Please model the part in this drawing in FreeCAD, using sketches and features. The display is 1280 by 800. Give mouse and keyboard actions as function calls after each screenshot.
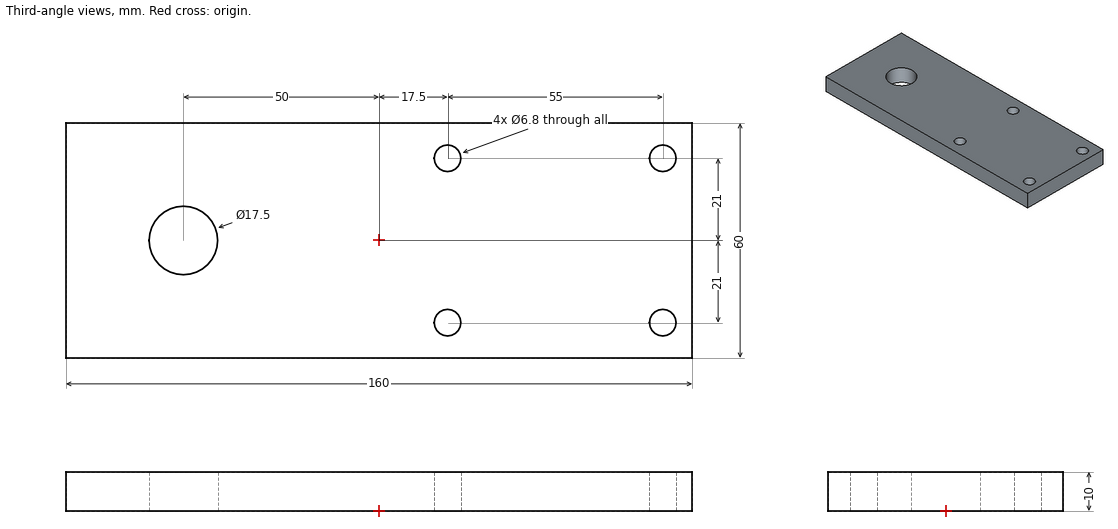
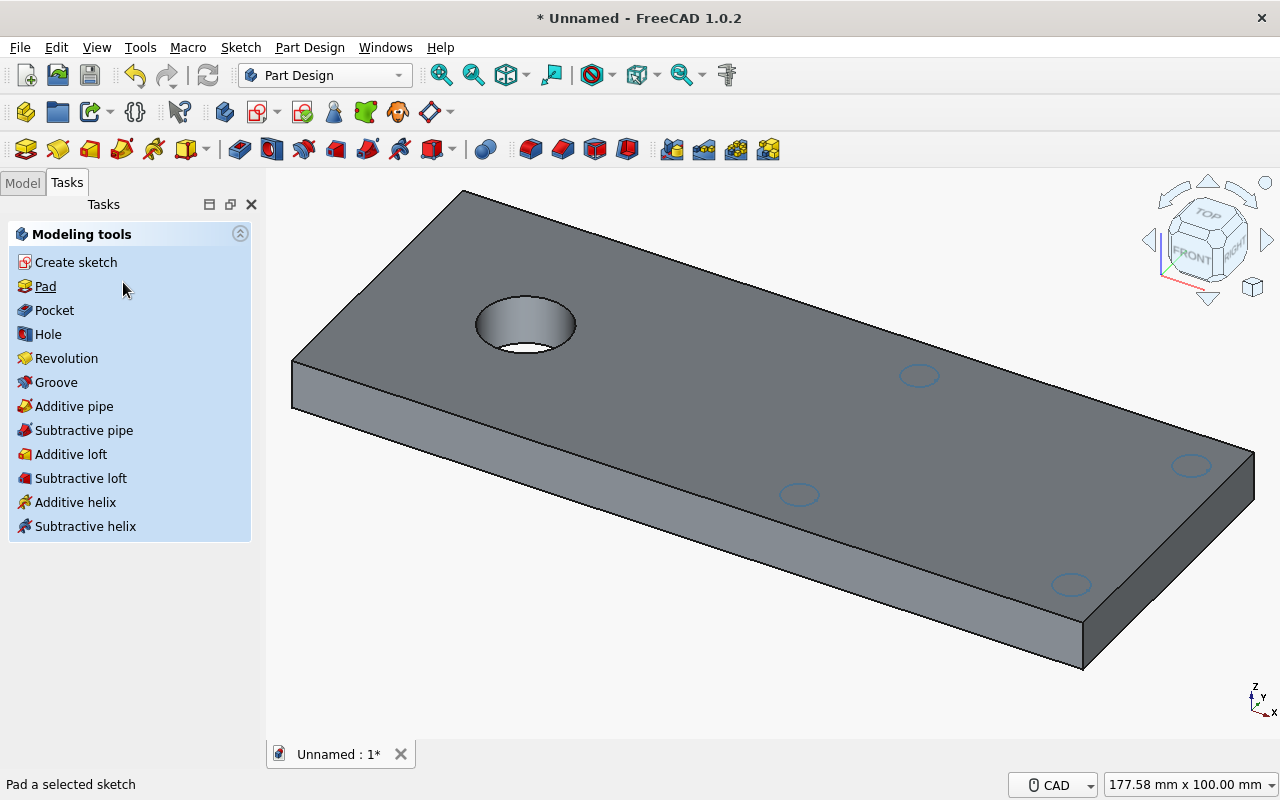
click(272, 150)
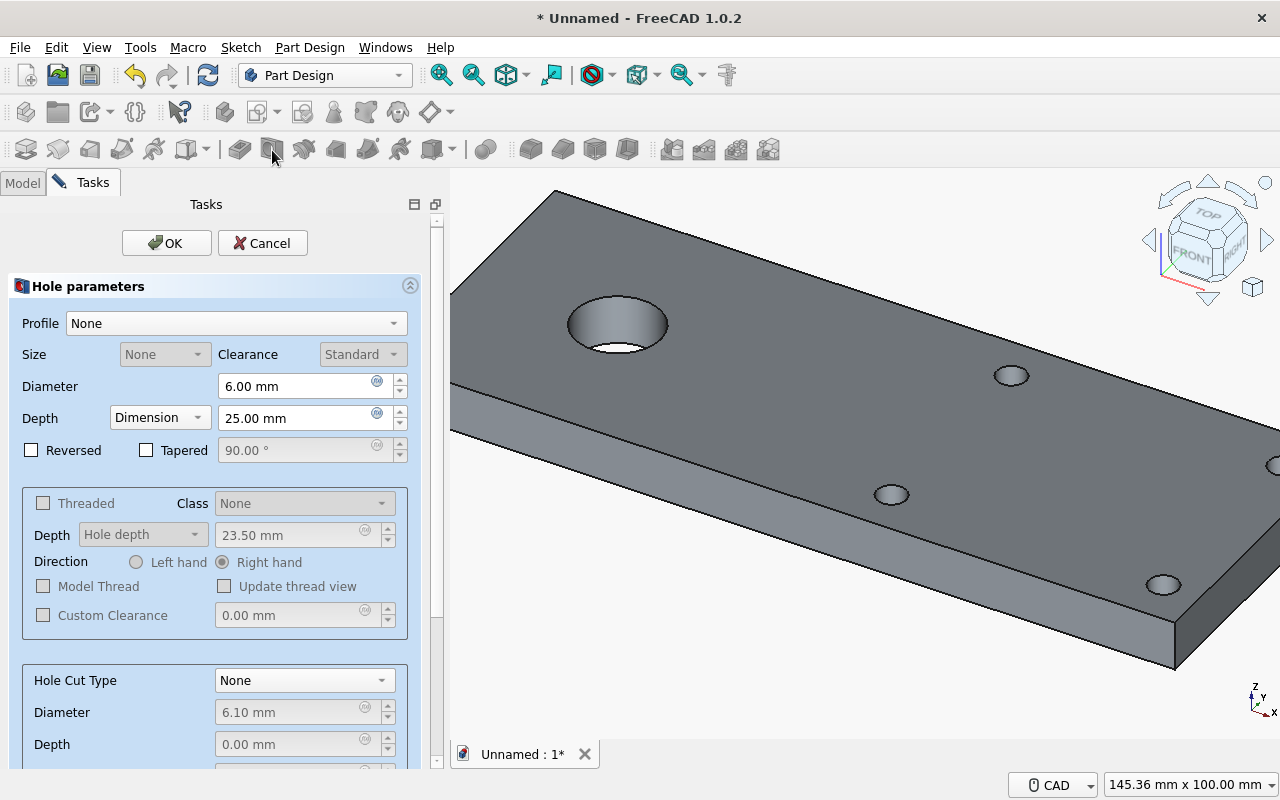
triple_click(305, 386)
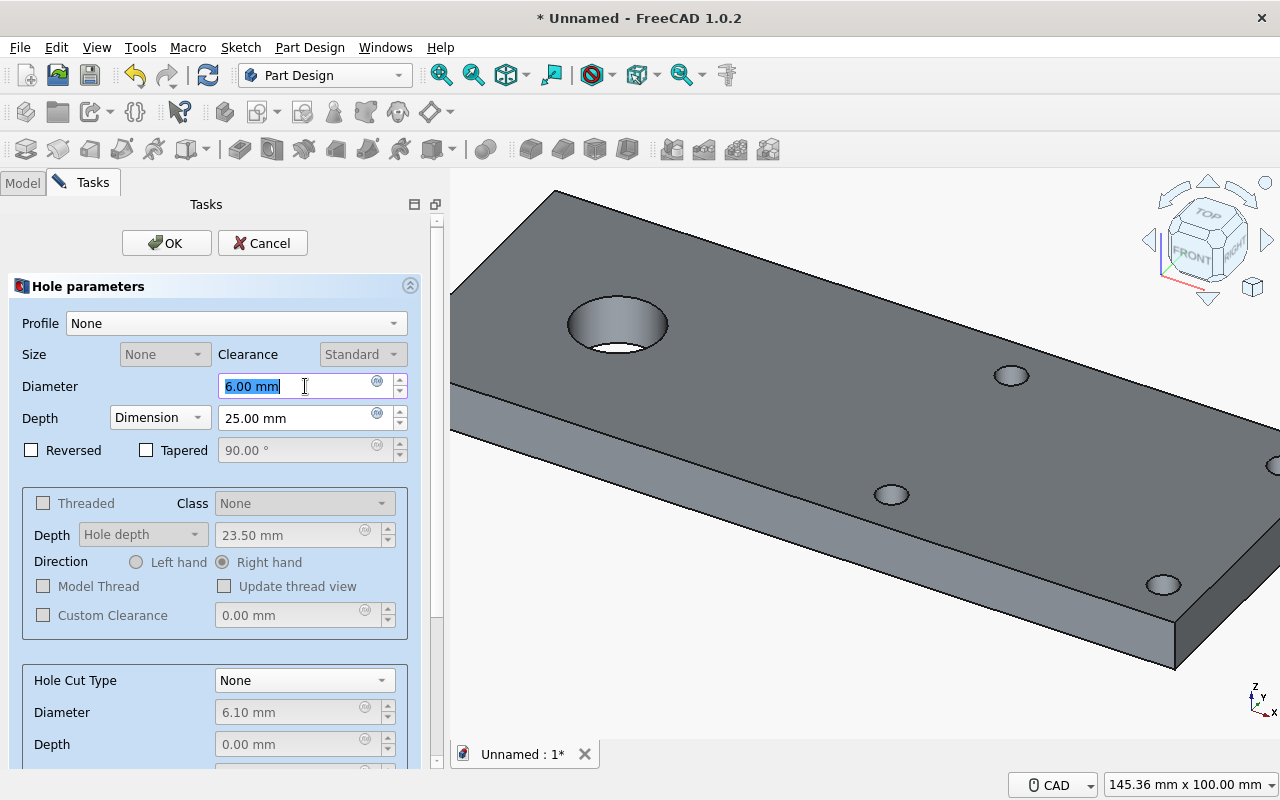
text(6.8)
key(Tab)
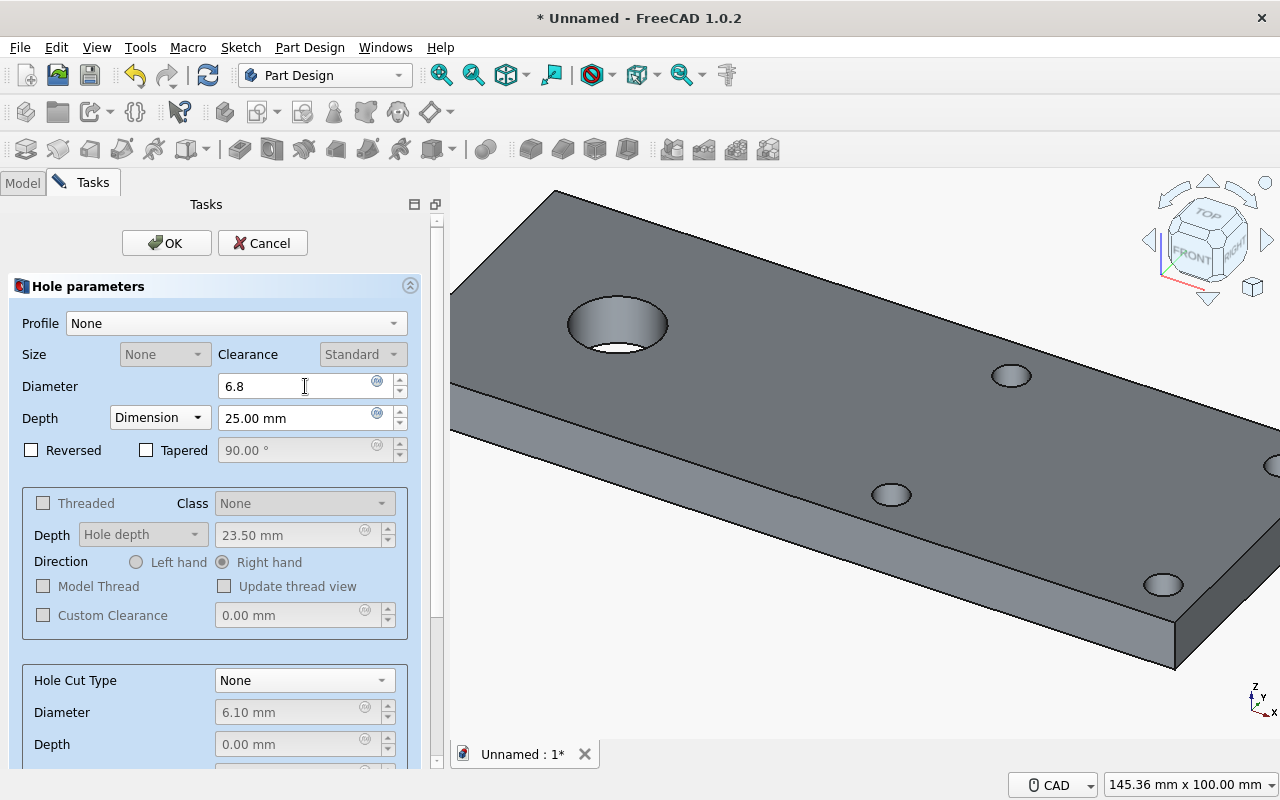
click(161, 418)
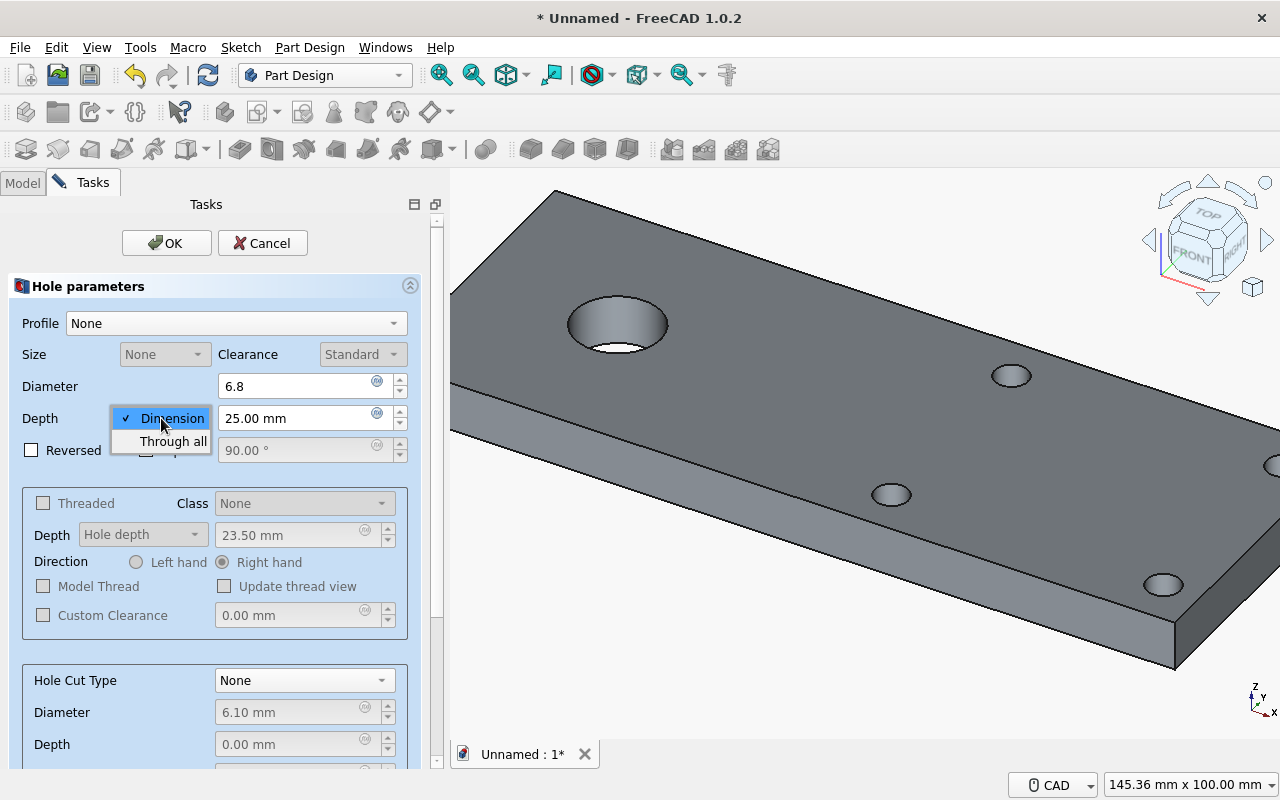
click(160, 442)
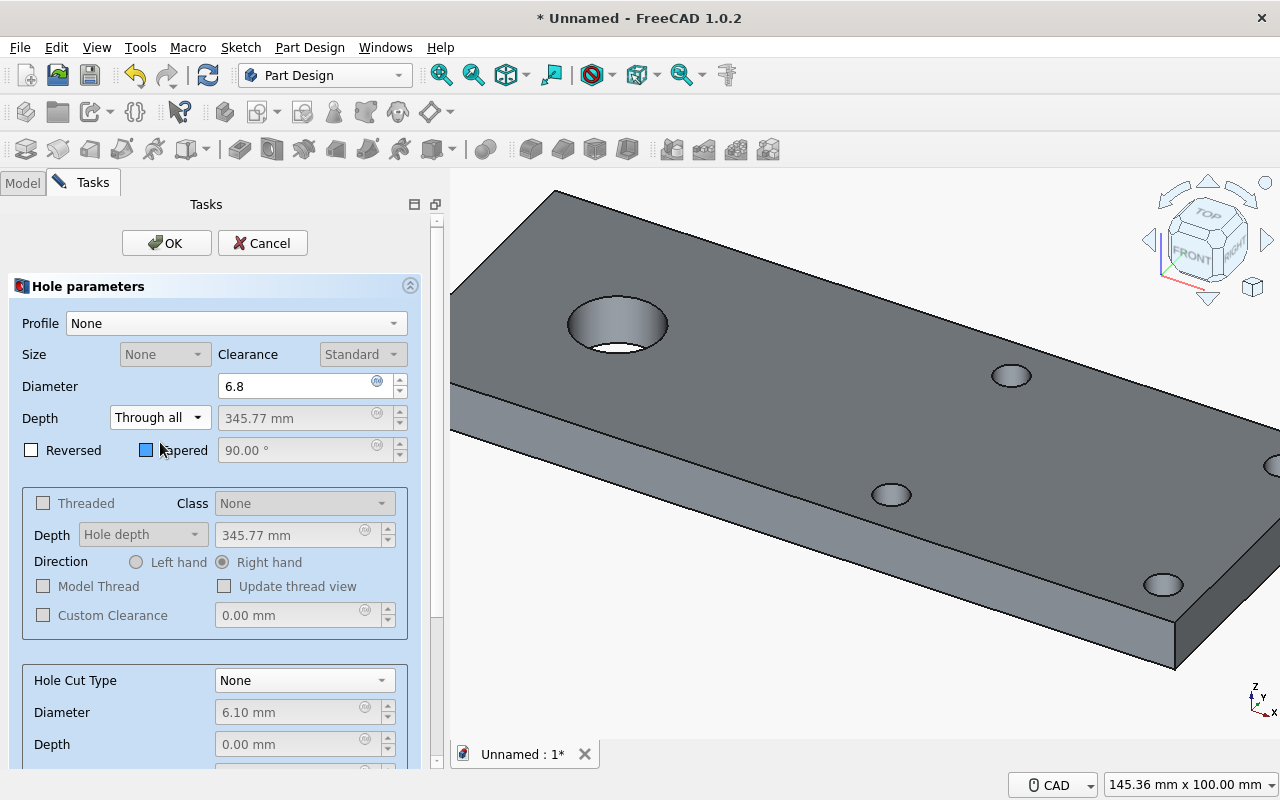
click(167, 243)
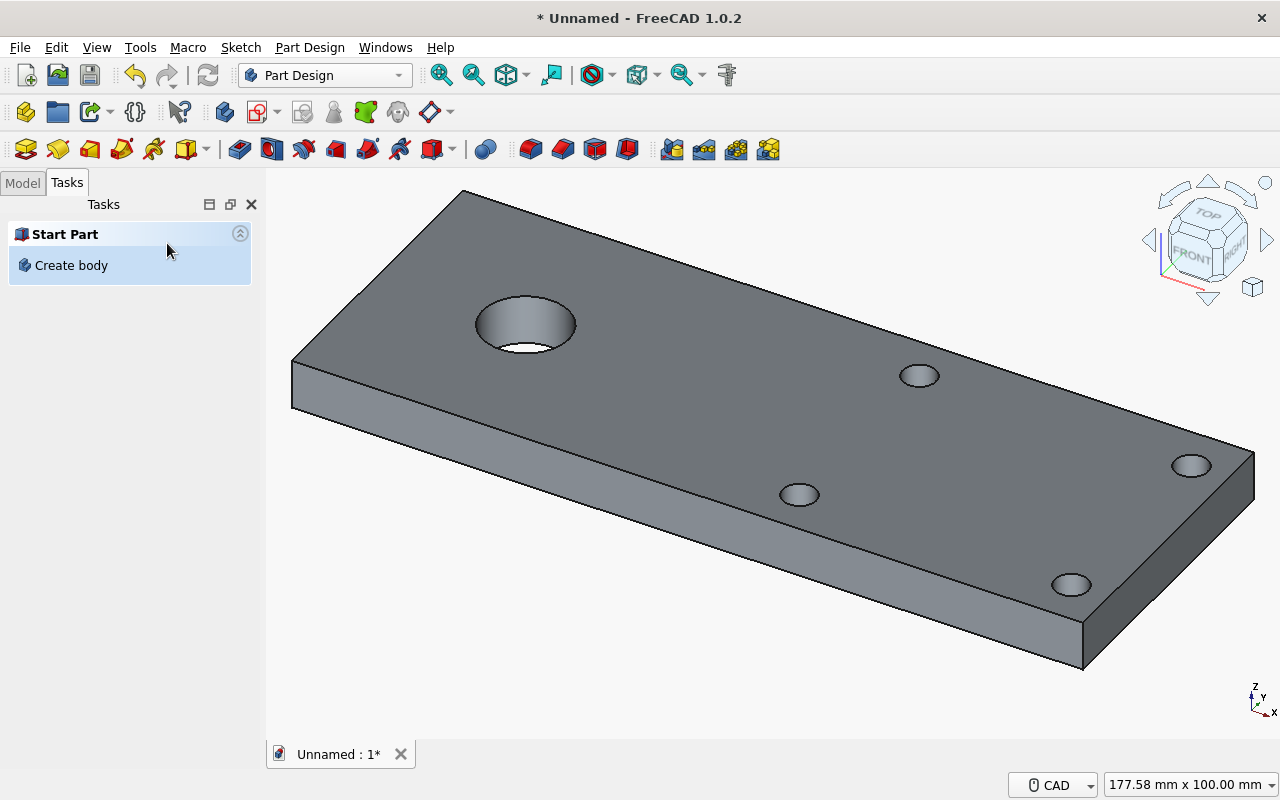
key(0)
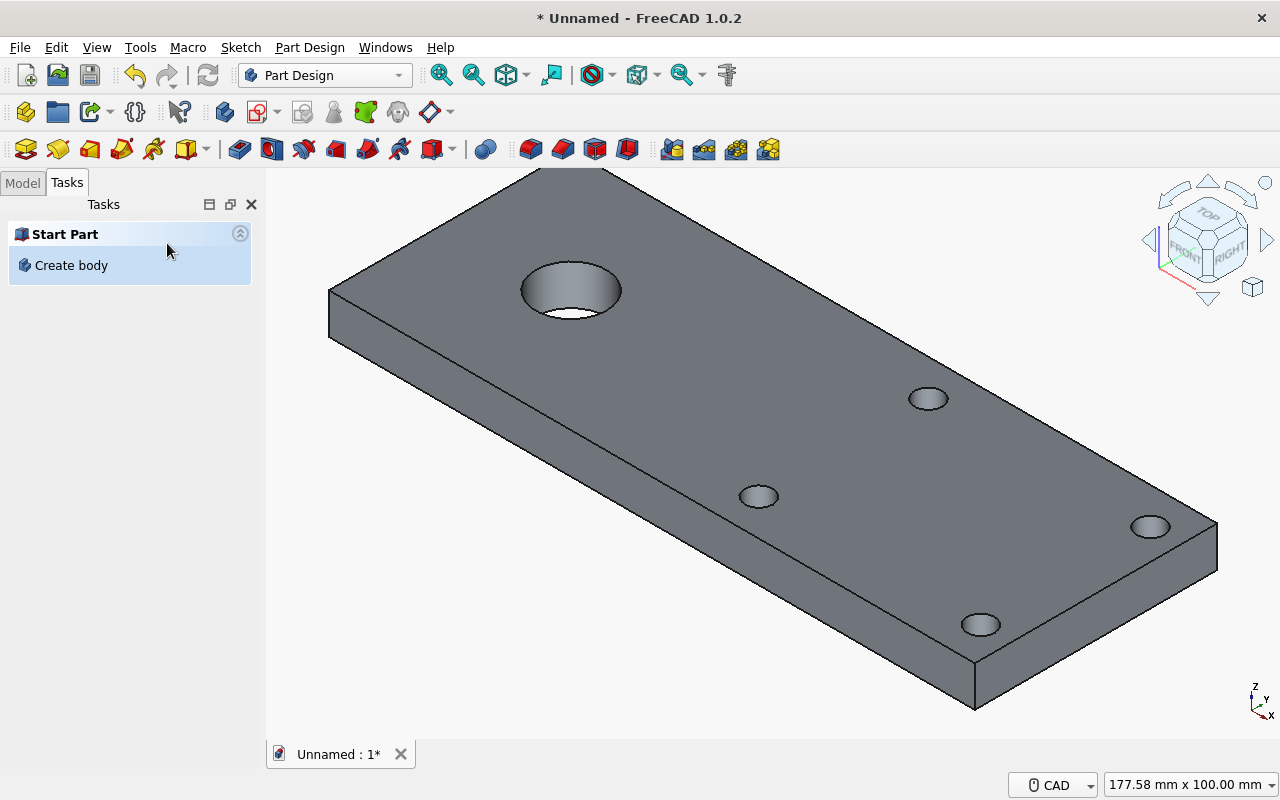
click(442, 76)